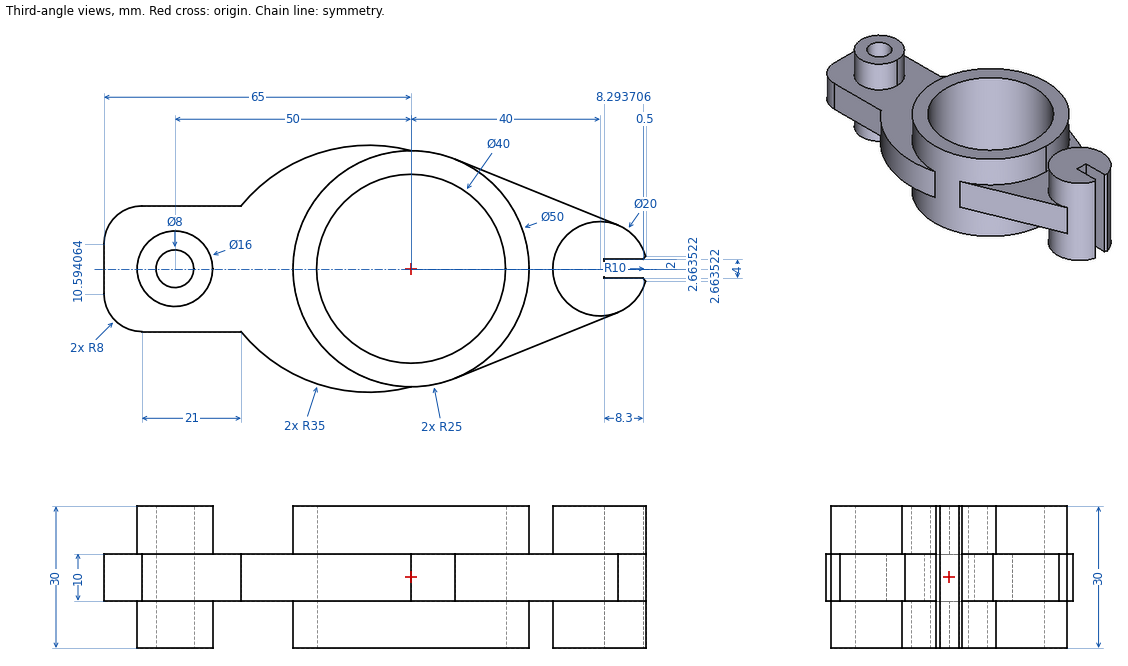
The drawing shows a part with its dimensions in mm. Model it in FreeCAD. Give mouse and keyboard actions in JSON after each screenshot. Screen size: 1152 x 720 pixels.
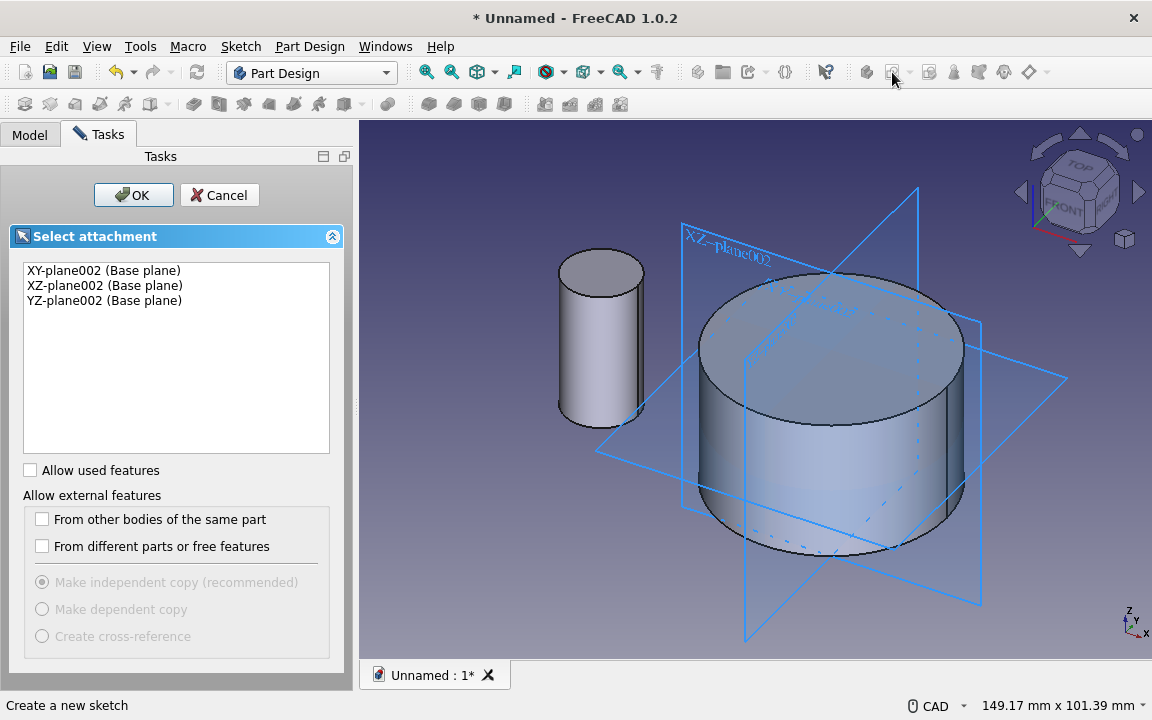
{"action": "left_click", "coordinate": [84, 270]}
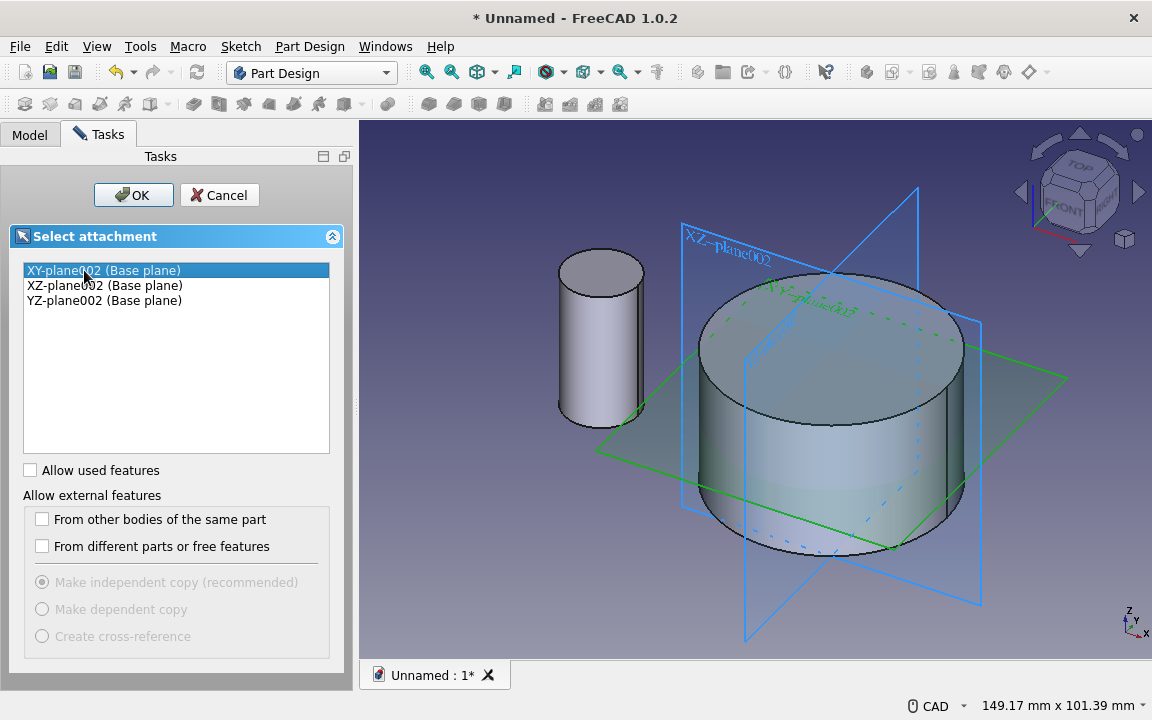
{"action": "left_click", "coordinate": [134, 195]}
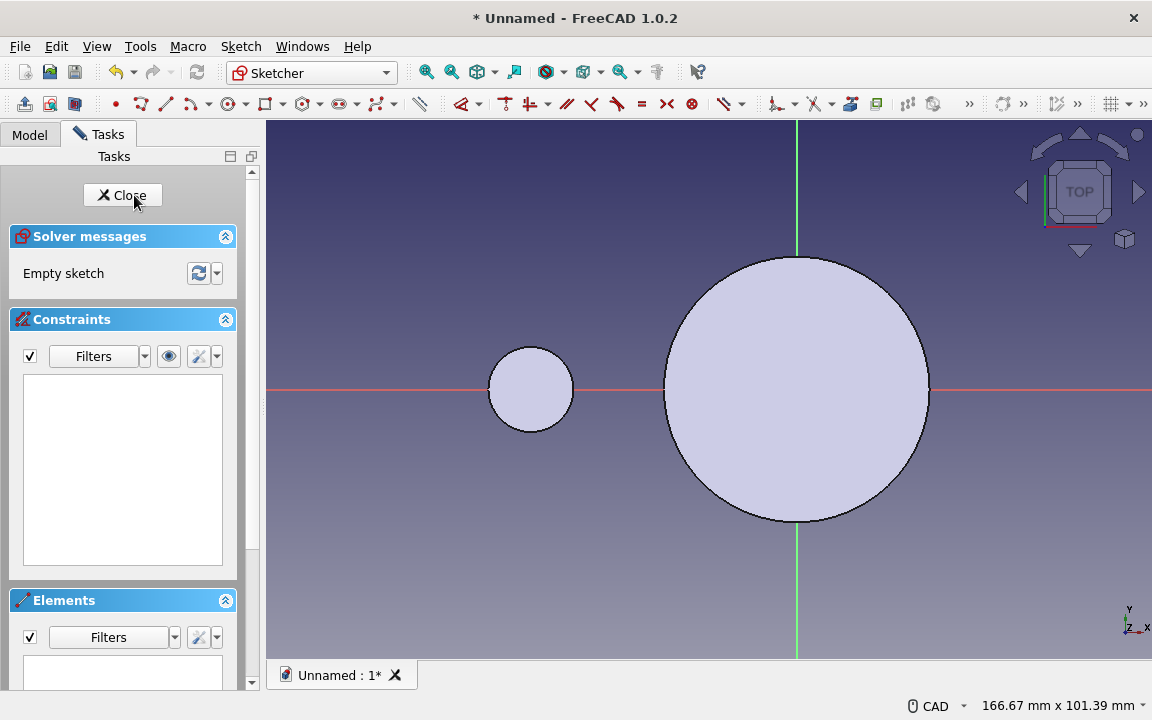
{"action": "scroll", "coordinate": [640, 390], "scroll_direction": "down", "scroll_amount": 5}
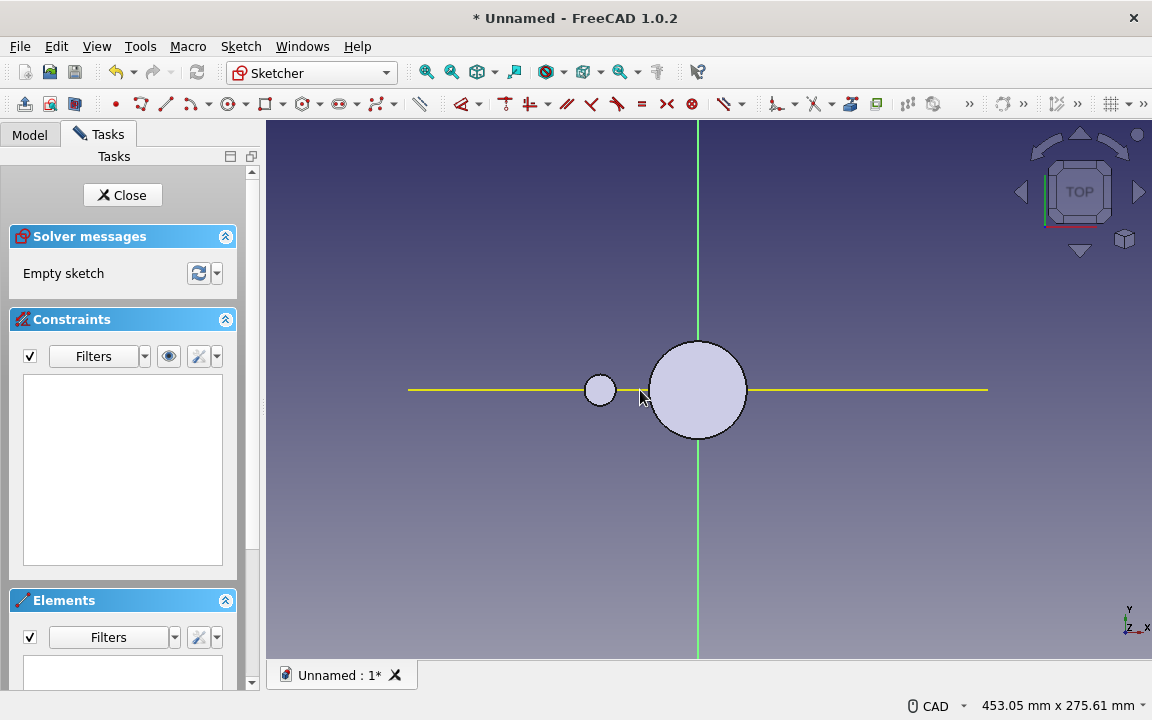
{"action": "scroll", "coordinate": [793, 390], "scroll_direction": "up", "scroll_amount": 11}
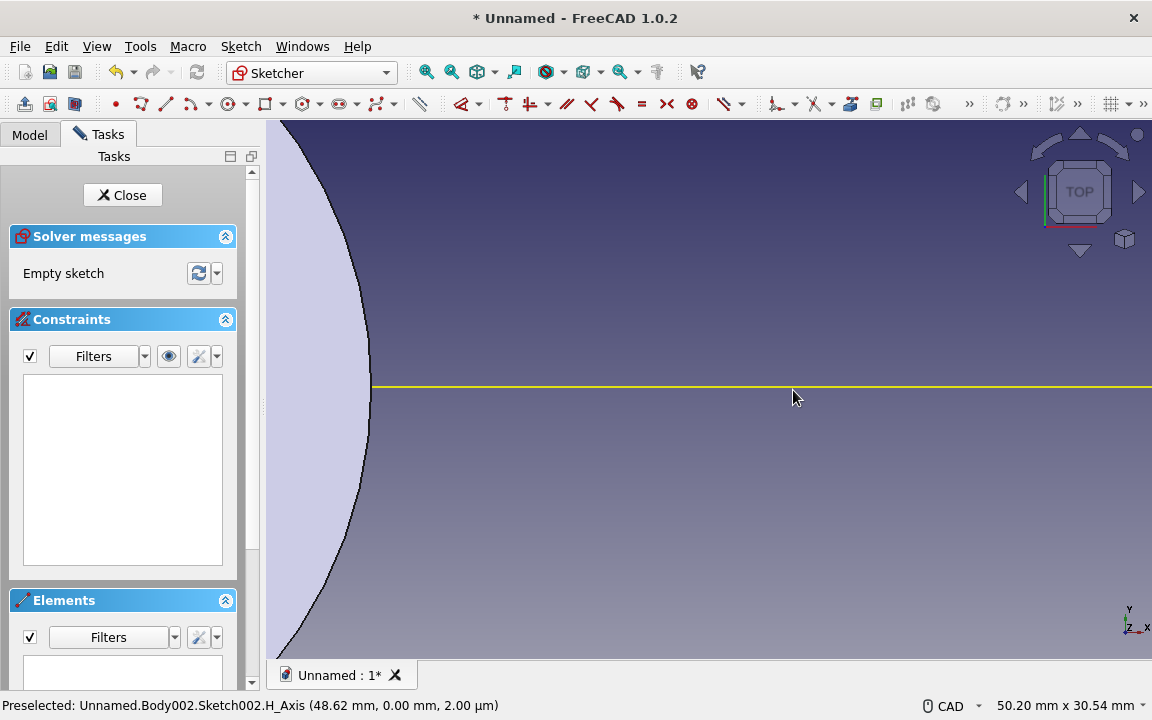
{"action": "left_click", "coordinate": [228, 104]}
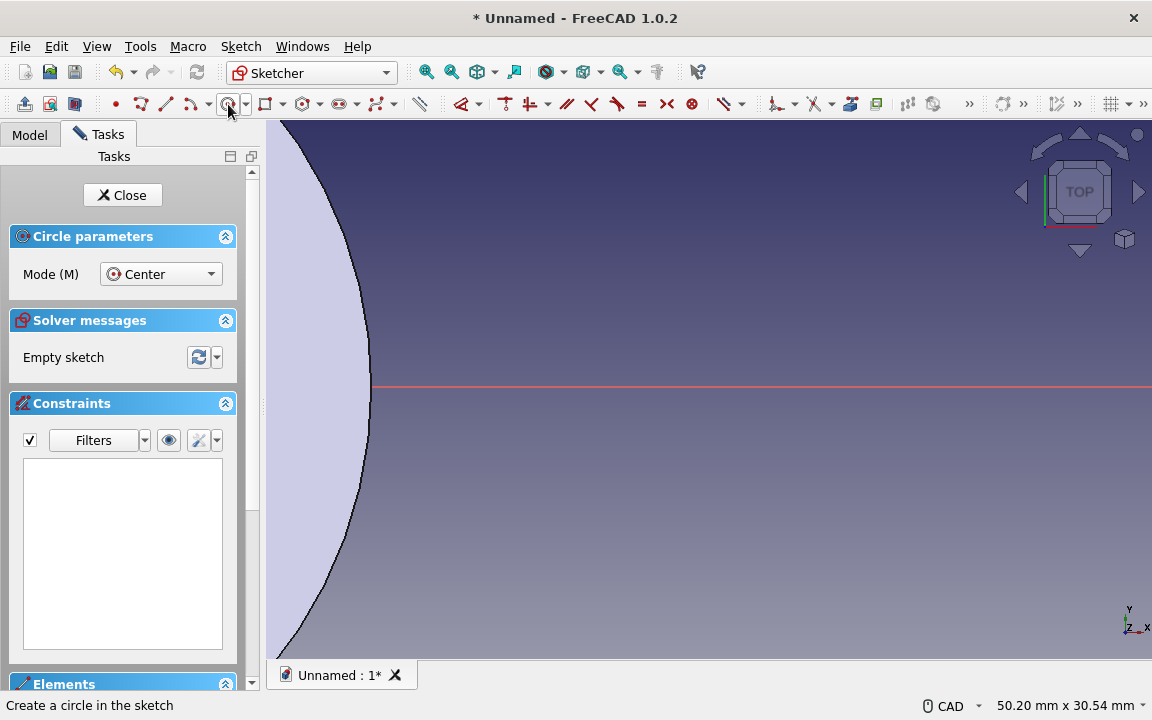
{"action": "left_click", "coordinate": [636, 387]}
{"action": "left_click", "coordinate": [761, 262]}
{"action": "key", "text": "Escape"}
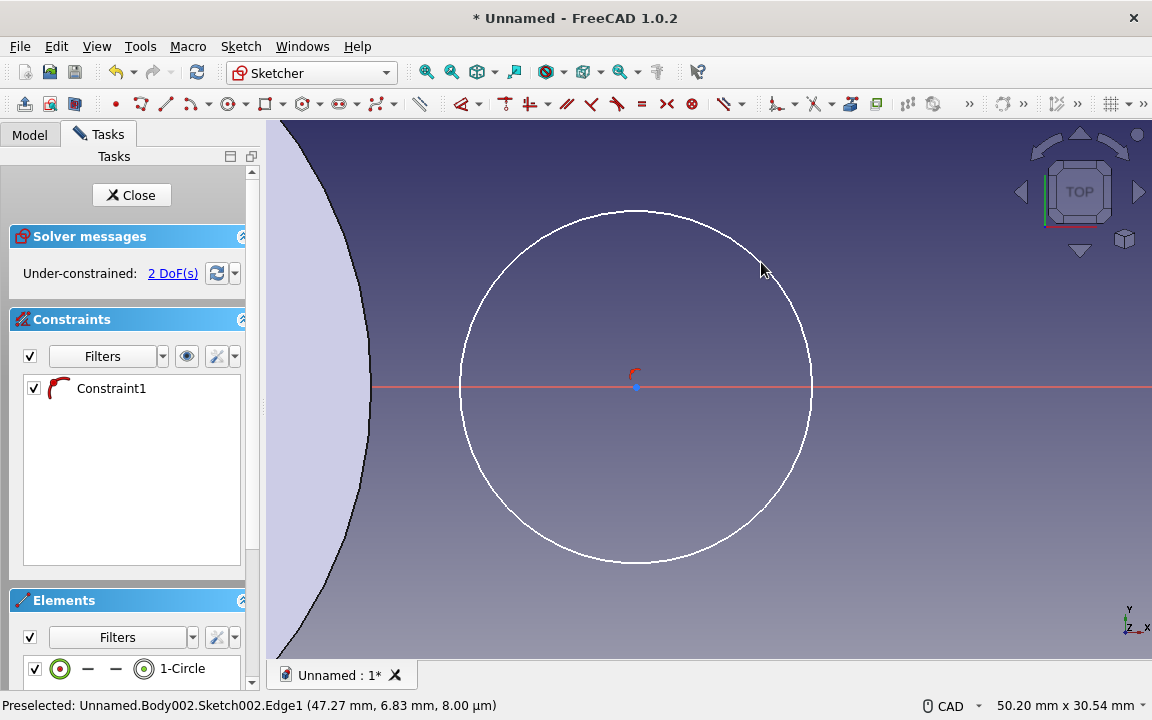
{"action": "left_click", "coordinate": [460, 104]}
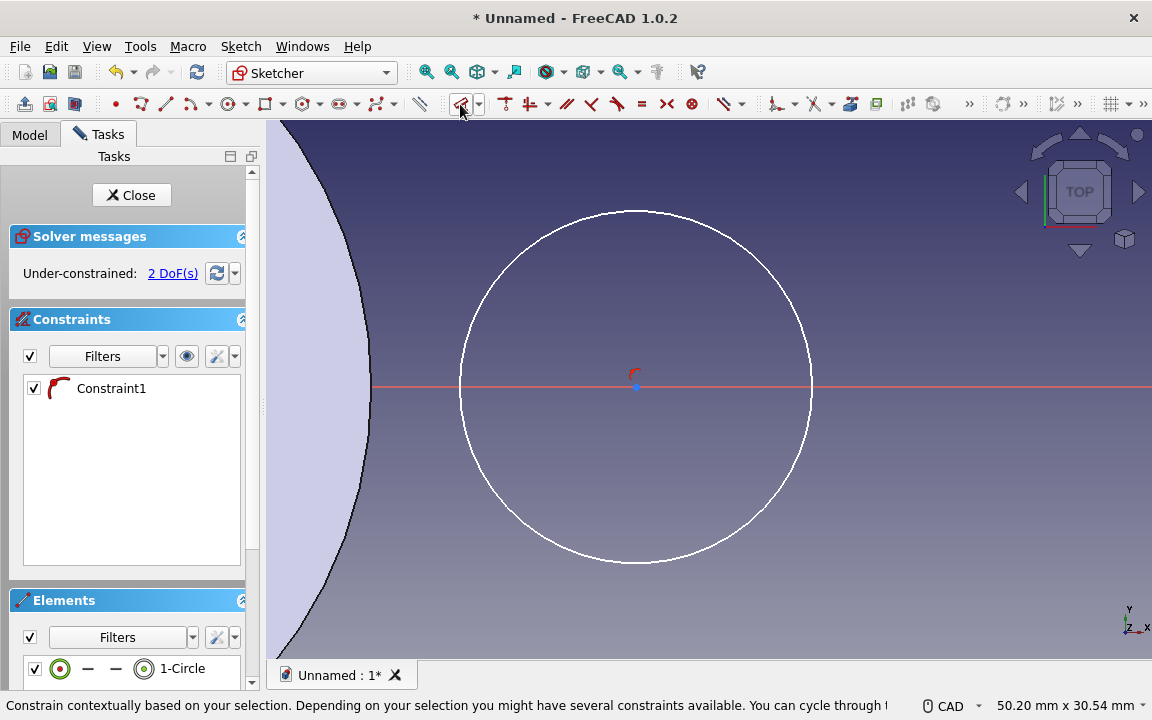
{"action": "left_click", "coordinate": [760, 262]}
{"action": "left_click", "coordinate": [783, 239]}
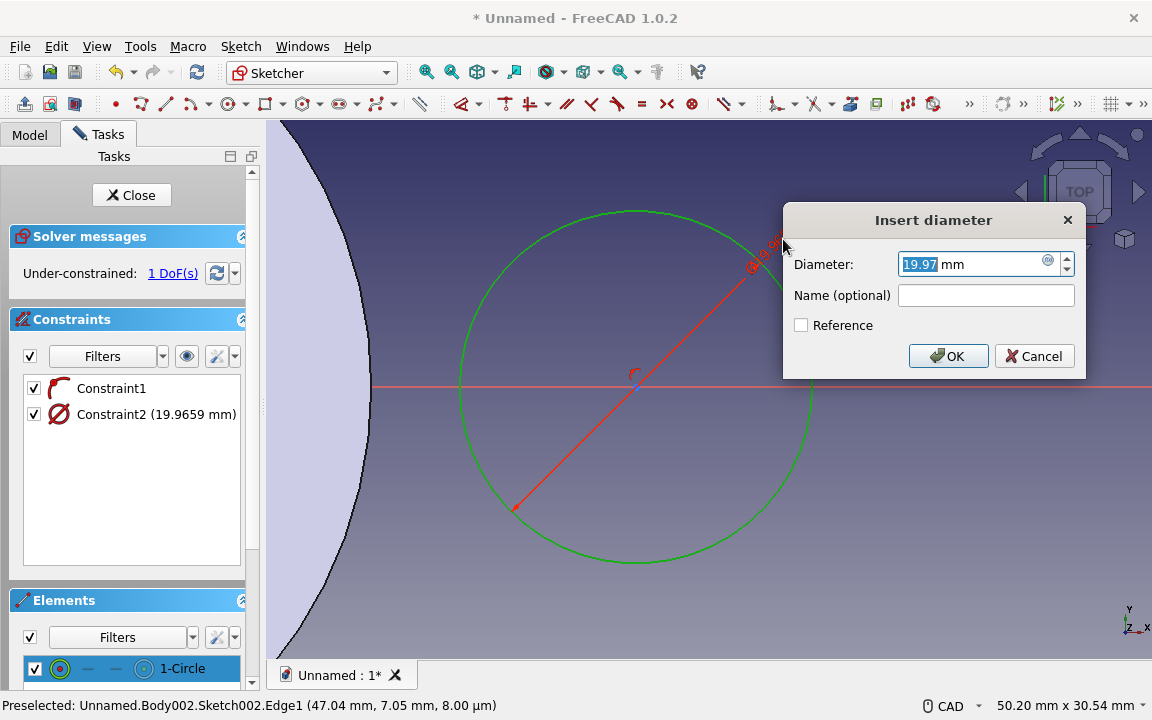
{"action": "type", "text": "20"}
{"action": "key", "text": "Return"}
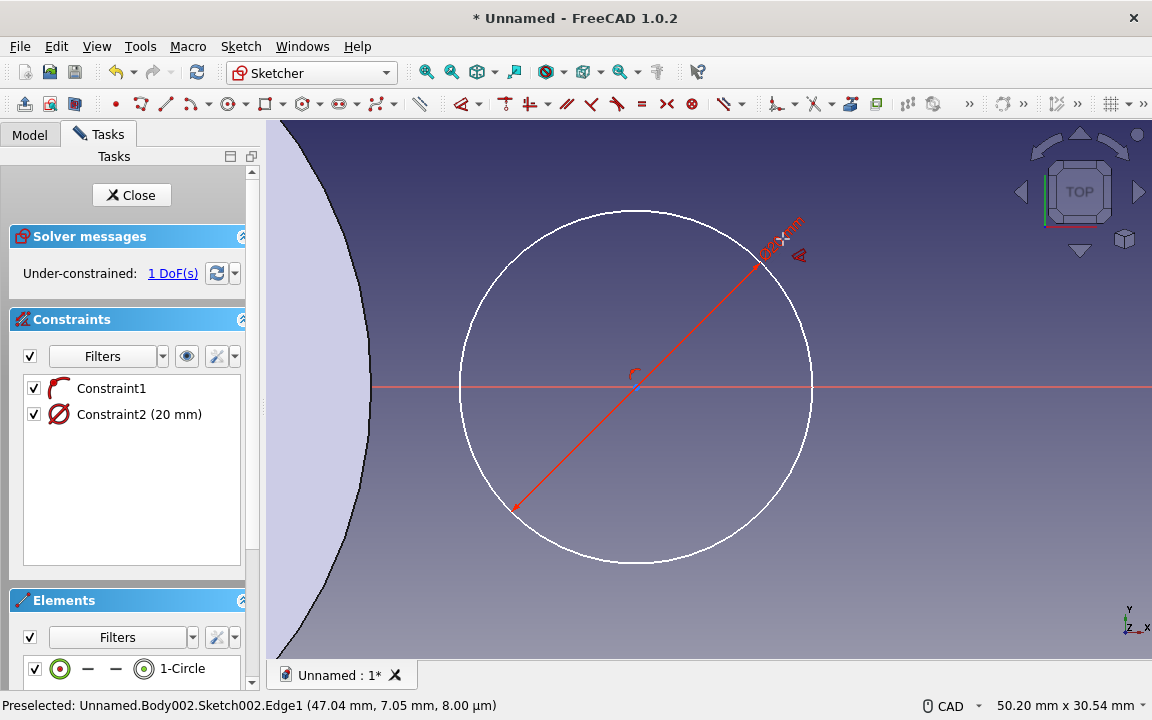
{"action": "left_click", "coordinate": [636, 387]}
{"action": "left_click", "coordinate": [386, 421]}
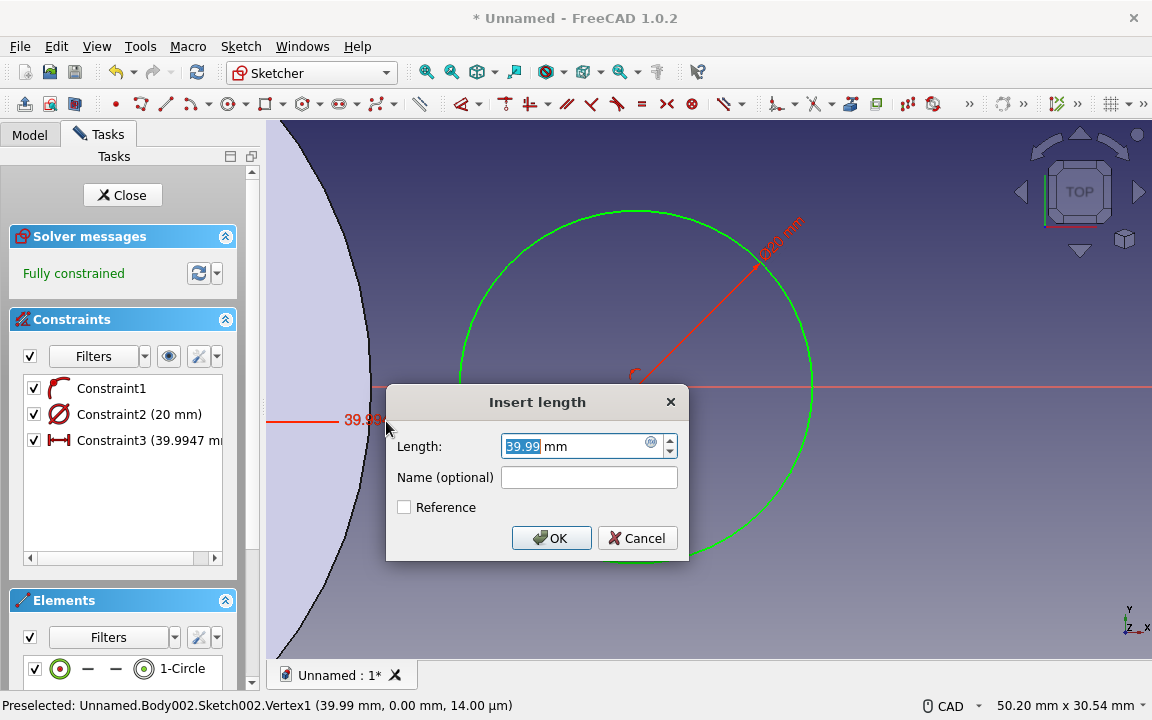
{"action": "type", "text": "40"}
{"action": "key", "text": "Return"}
{"action": "key", "text": "Escape"}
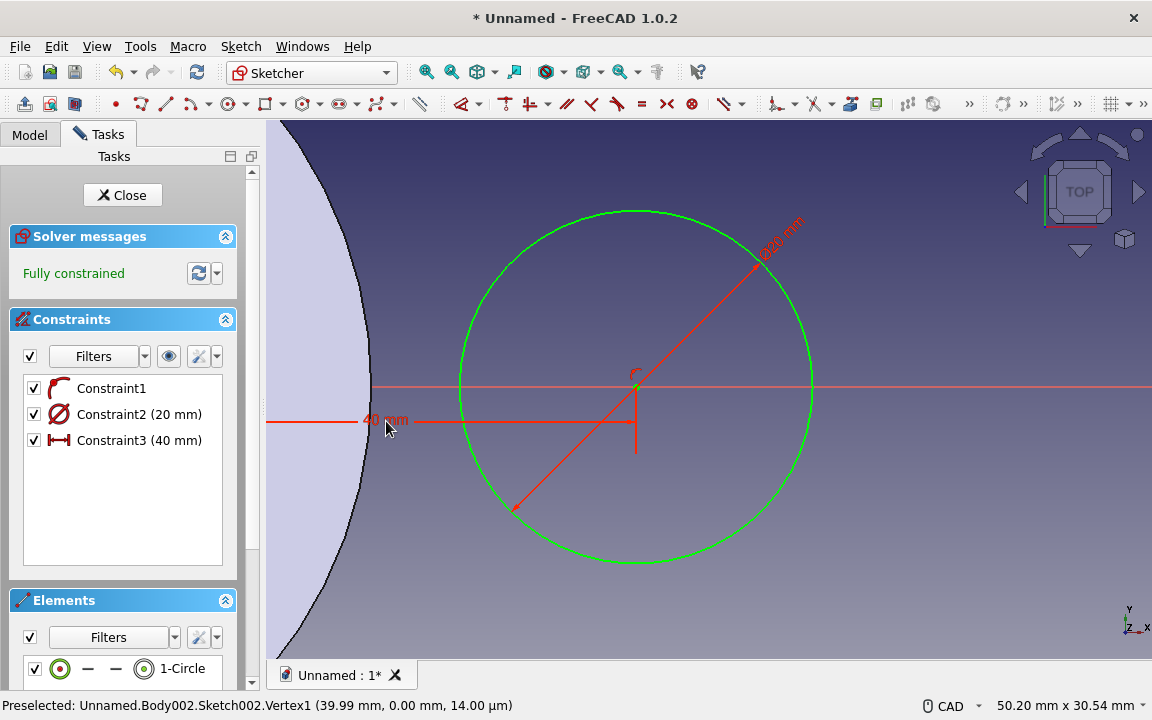
{"action": "left_click", "coordinate": [123, 195]}